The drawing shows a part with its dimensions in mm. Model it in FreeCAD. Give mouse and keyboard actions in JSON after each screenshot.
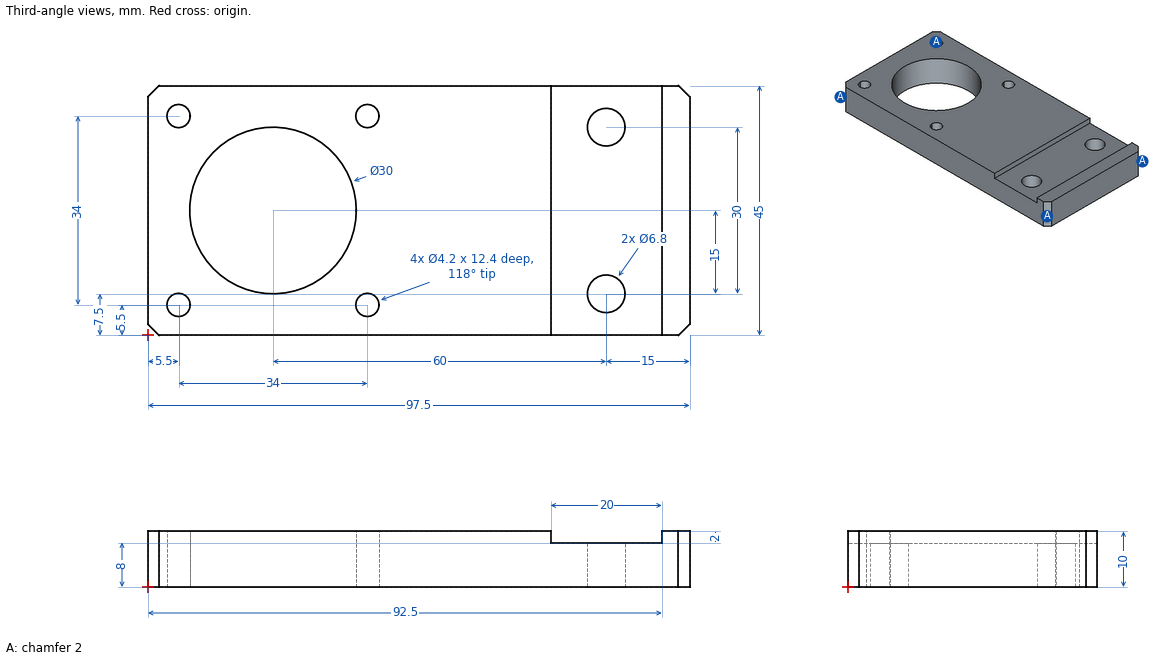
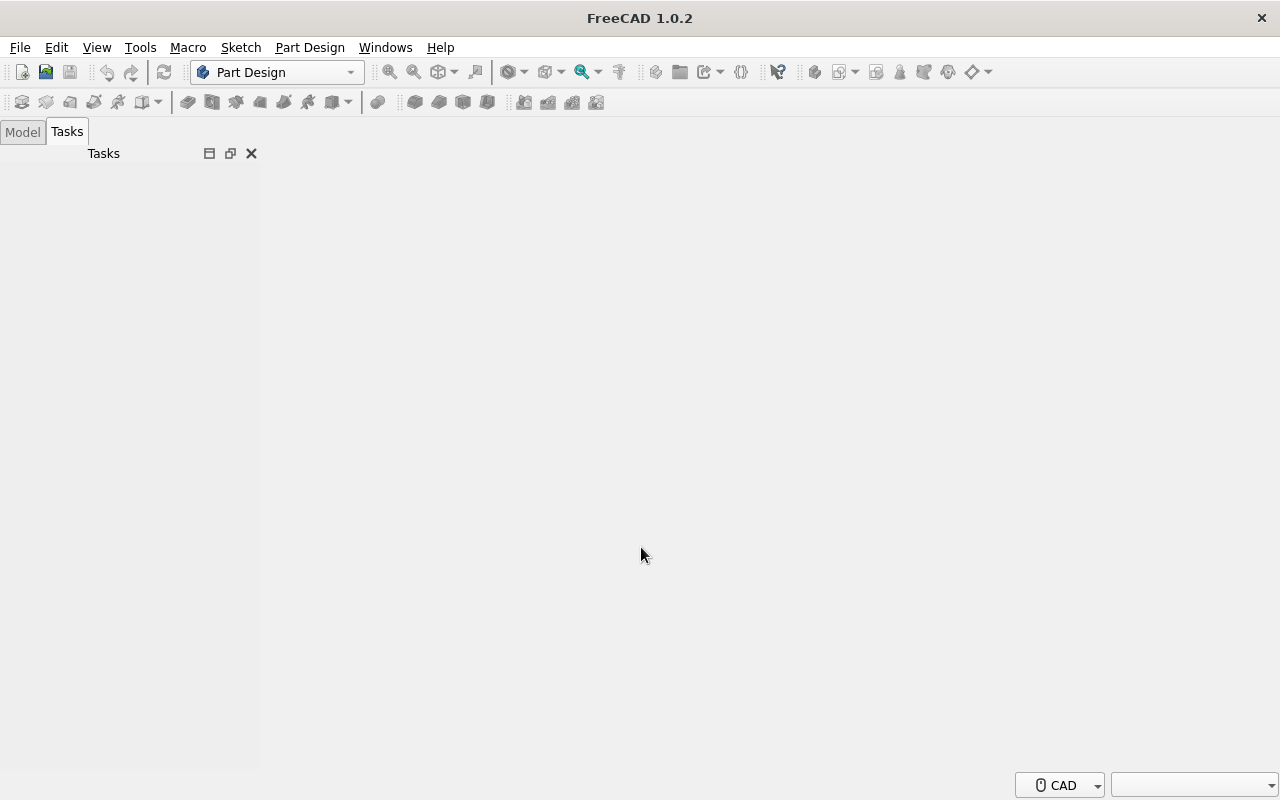
{"action": "key", "text": "ctrl+n"}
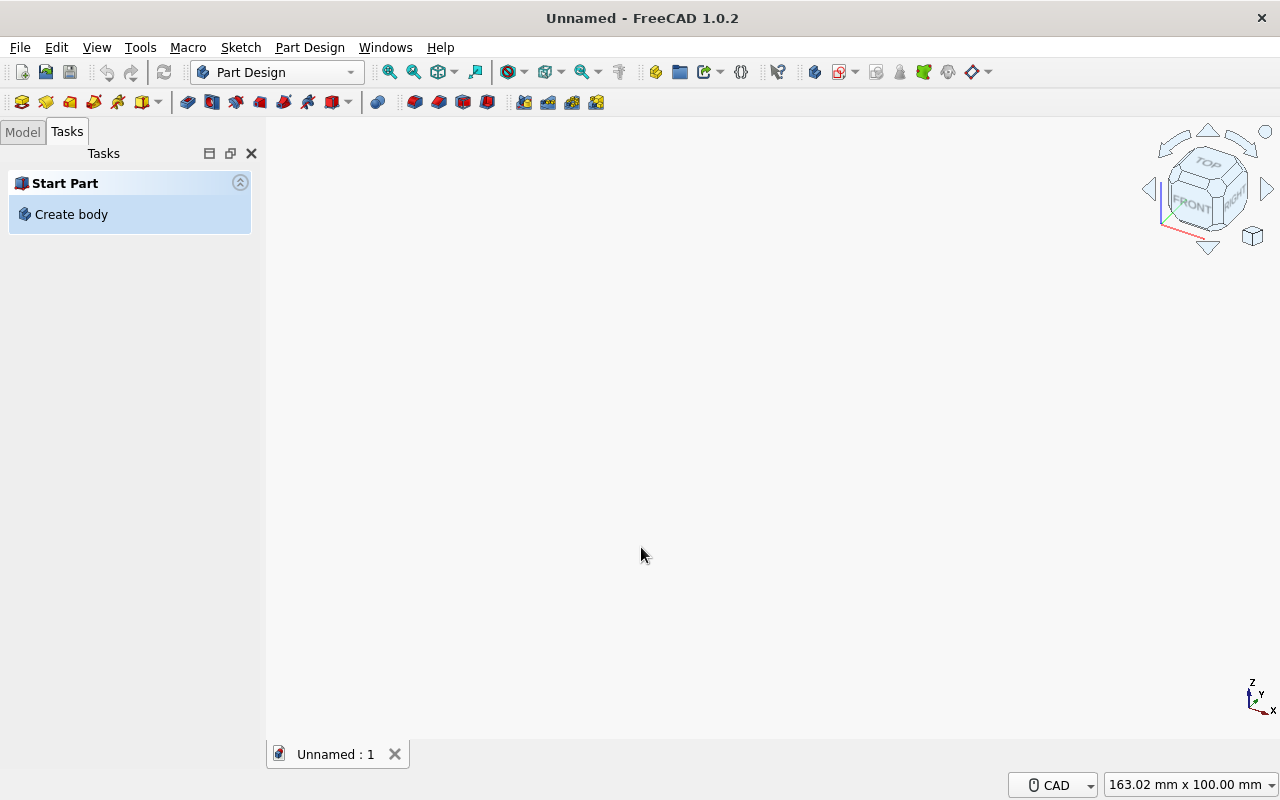
{"action": "left_click", "coordinate": [840, 72]}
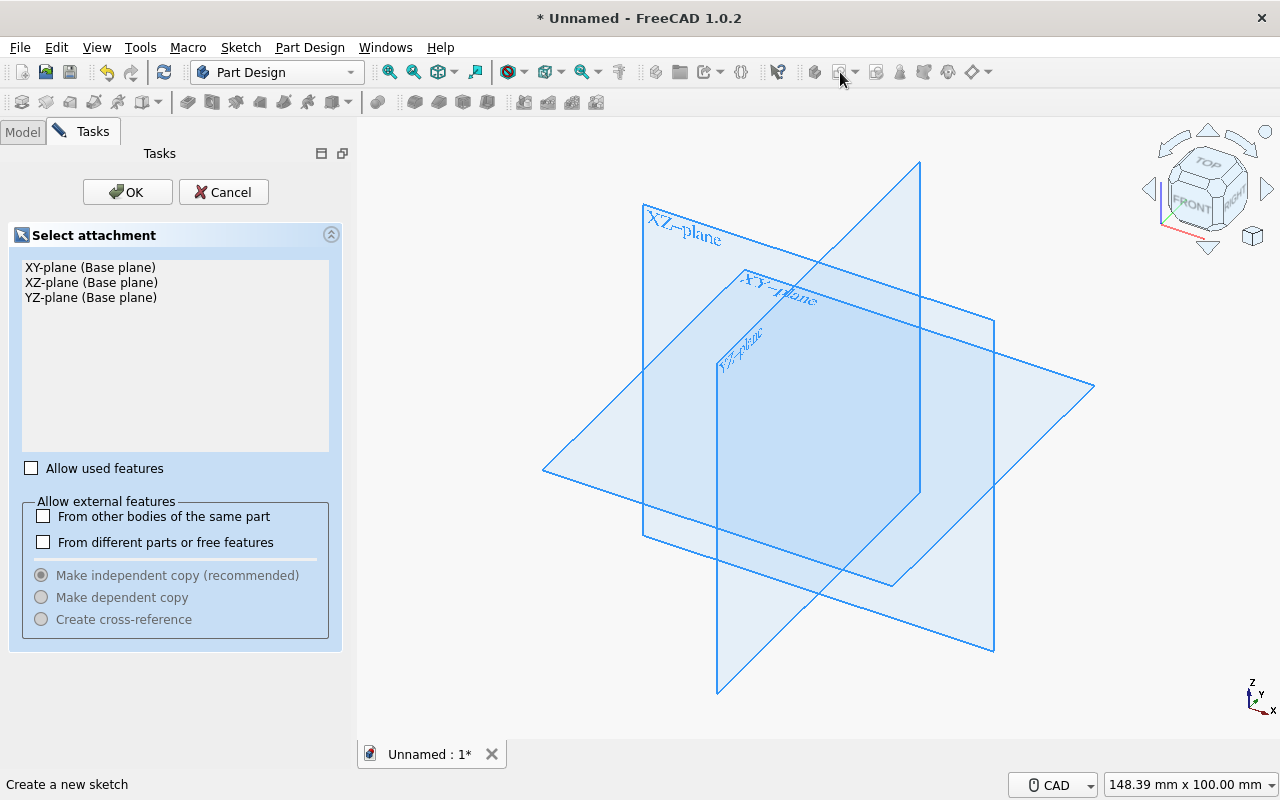
{"action": "left_click", "coordinate": [82, 268]}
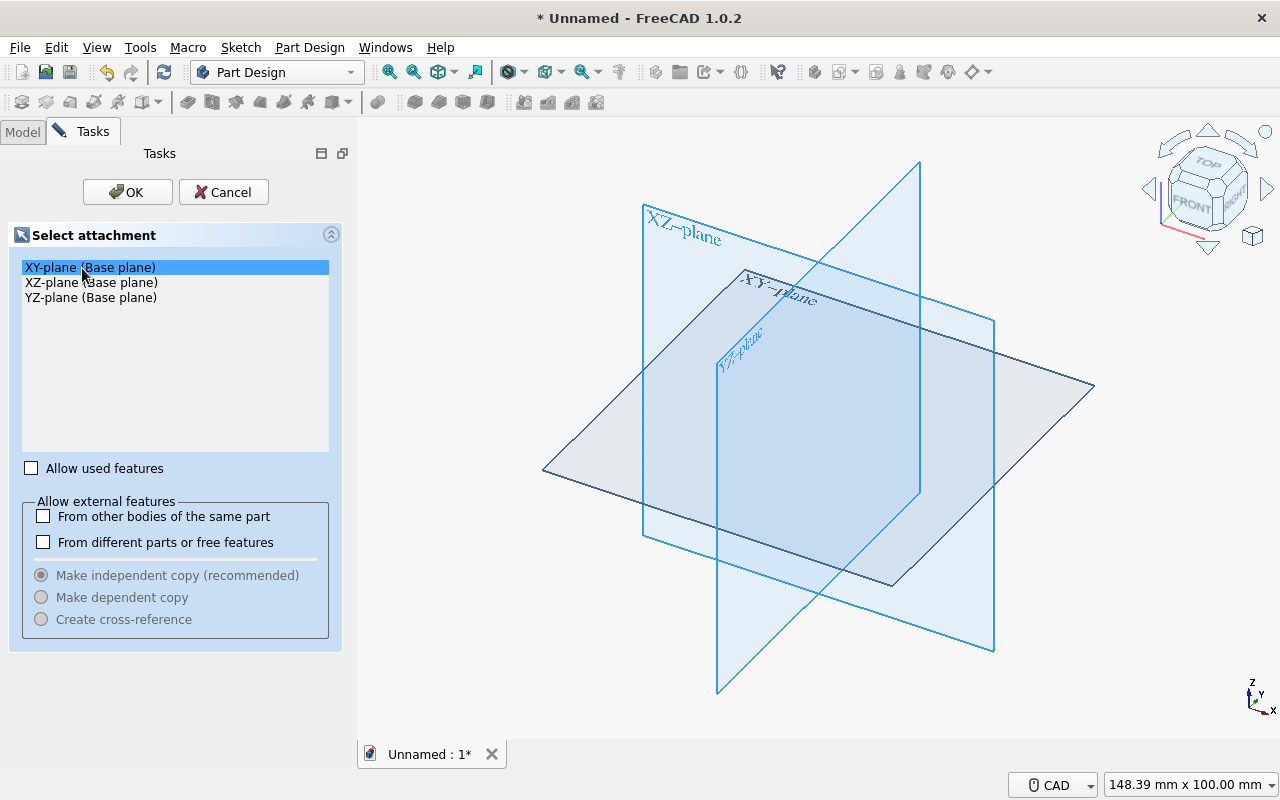
{"action": "left_click", "coordinate": [128, 192]}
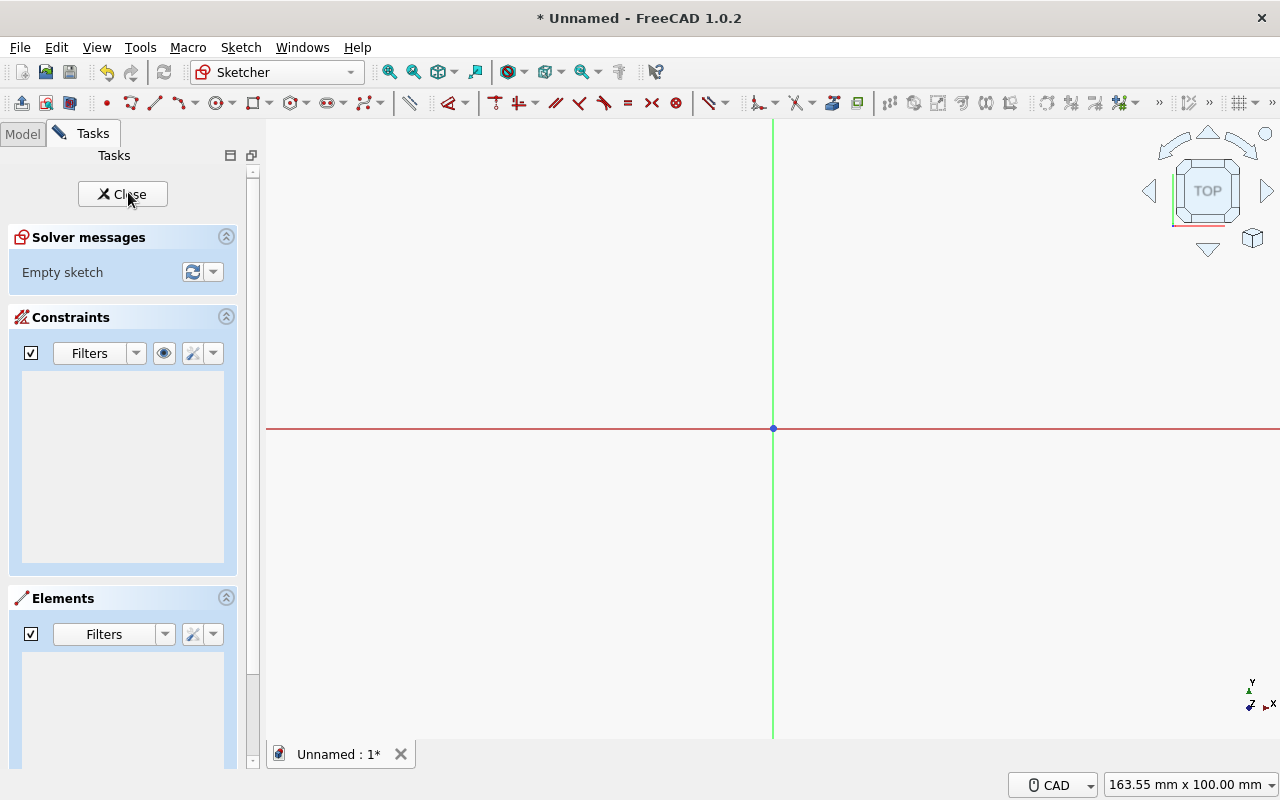
{"action": "scroll", "coordinate": [294, 711], "scroll_direction": "down", "scroll_amount": 2}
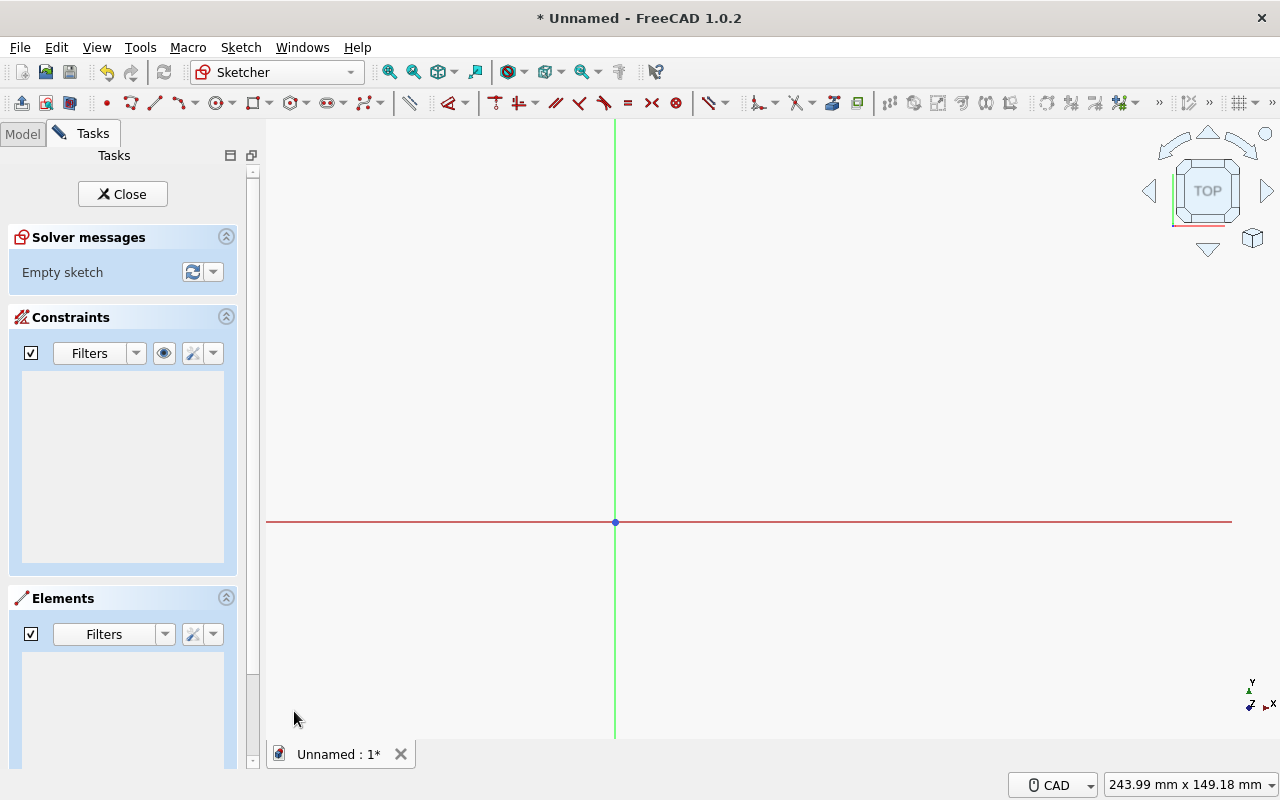
{"action": "scroll", "coordinate": [1048, 428], "scroll_direction": "up", "scroll_amount": 2}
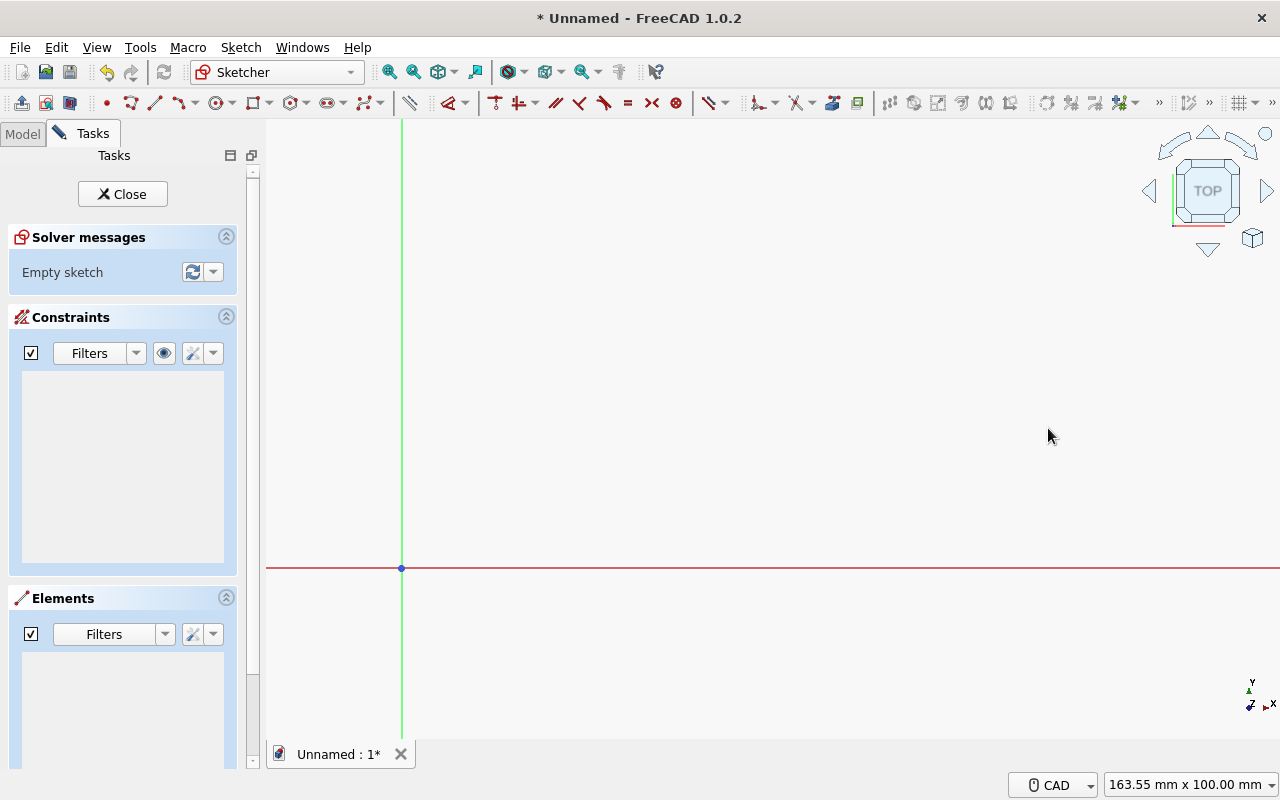
{"action": "left_click", "coordinate": [254, 104]}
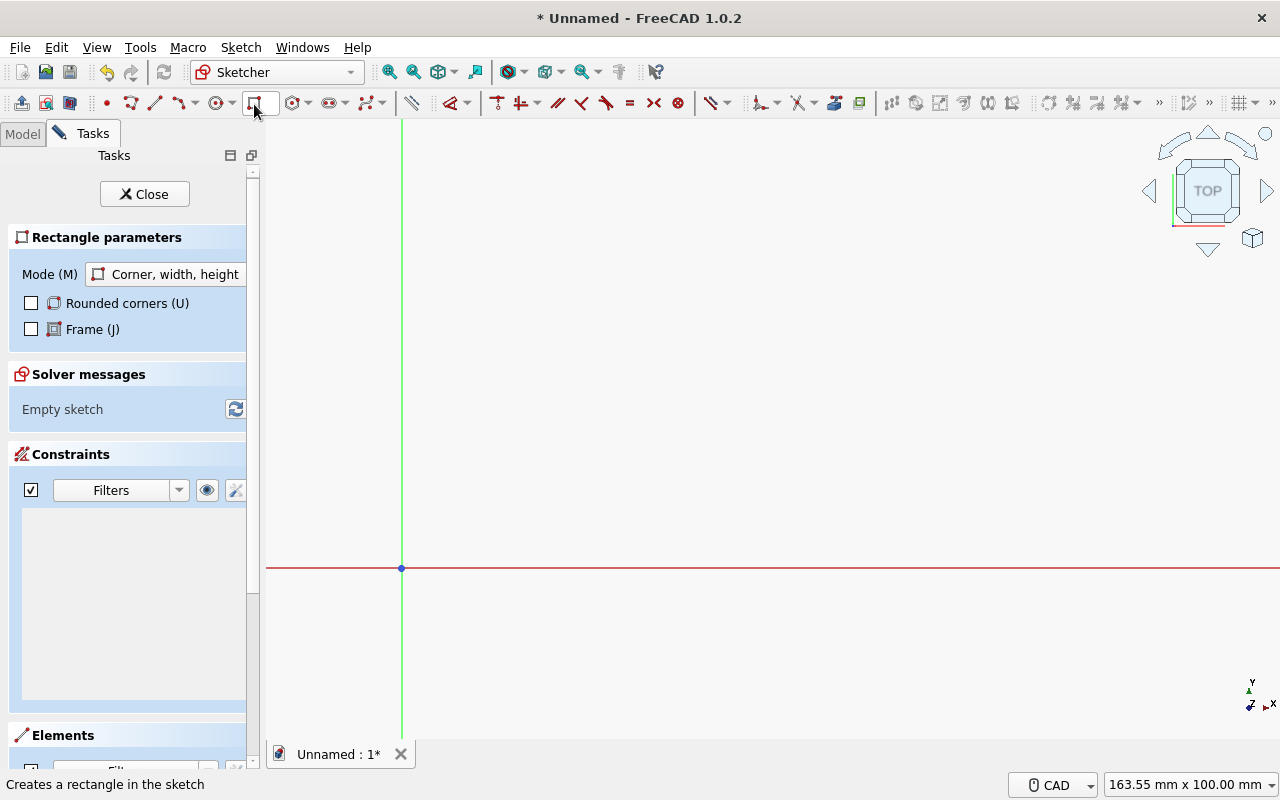
{"action": "left_click", "coordinate": [402, 568]}
{"action": "left_click", "coordinate": [1006, 289]}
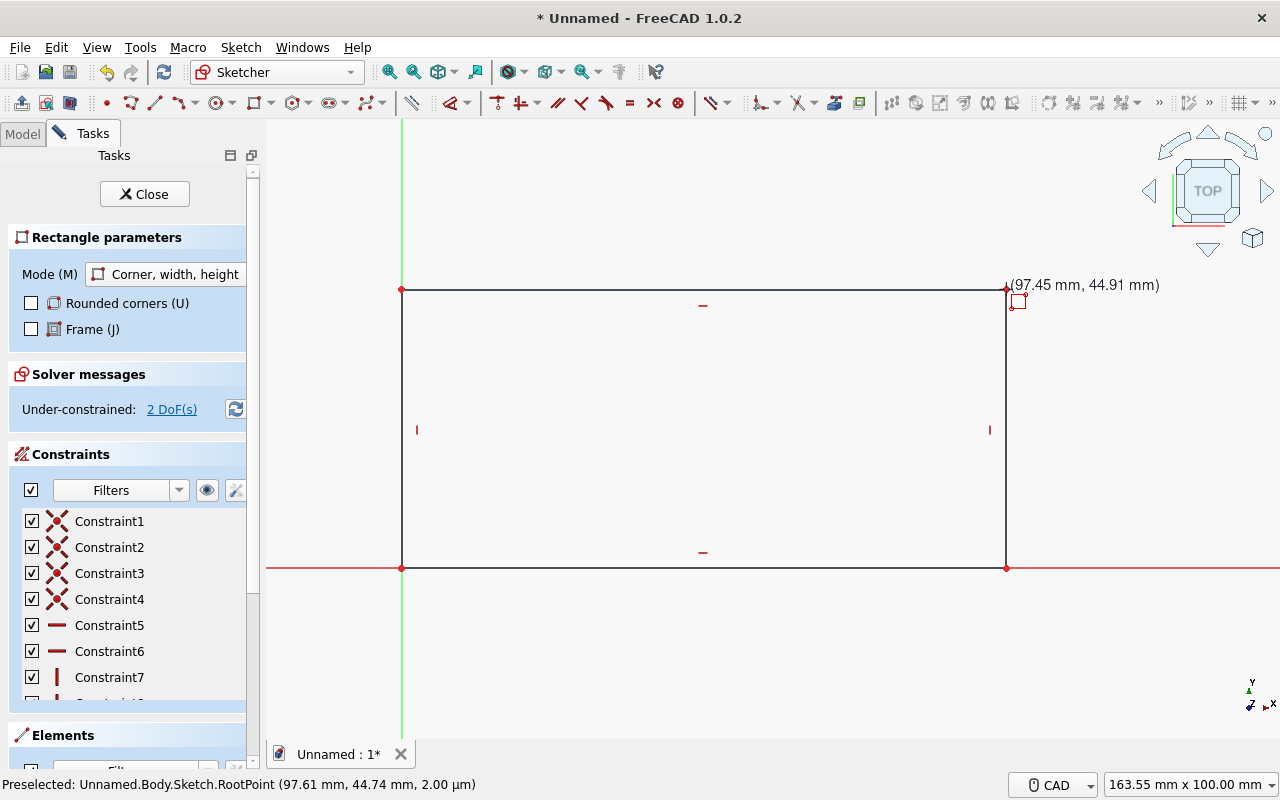
{"action": "key", "text": "g c"}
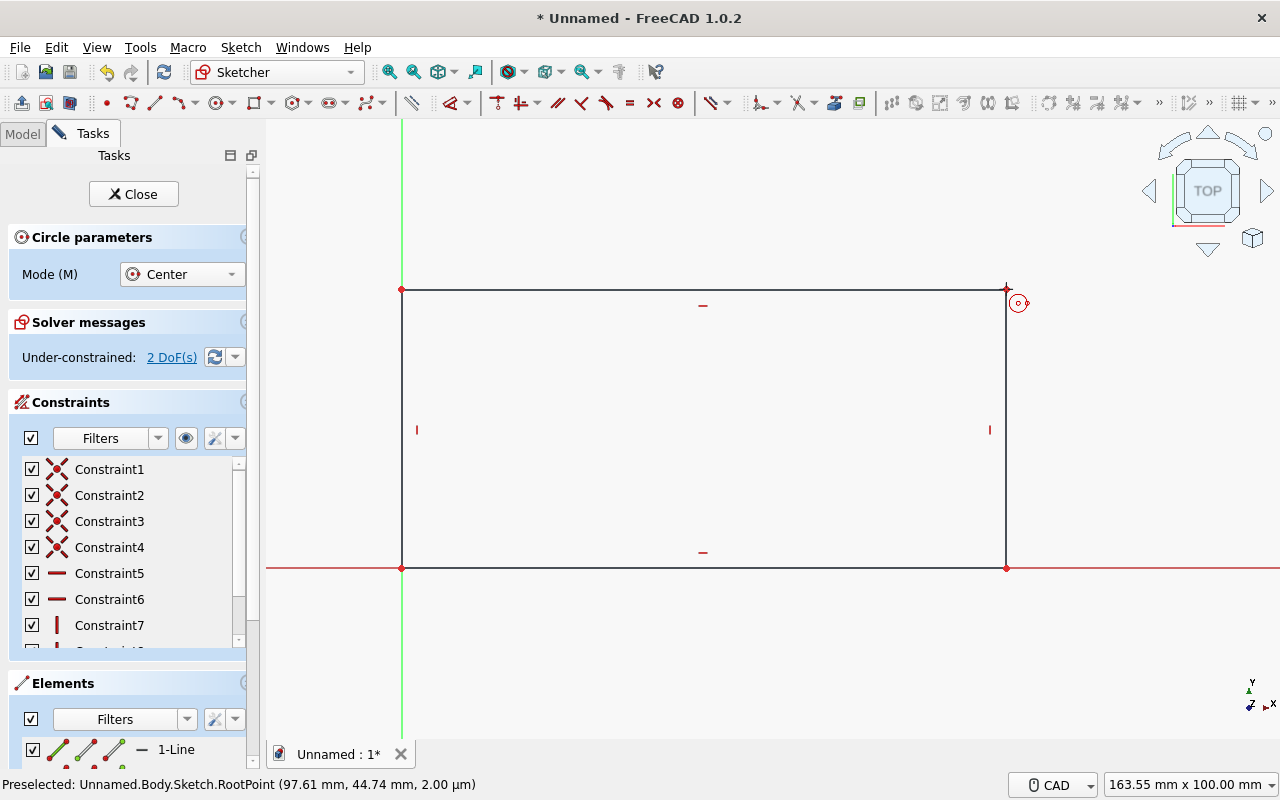
{"action": "left_click", "coordinate": [913, 522]}
{"action": "left_click", "coordinate": [928, 507]}